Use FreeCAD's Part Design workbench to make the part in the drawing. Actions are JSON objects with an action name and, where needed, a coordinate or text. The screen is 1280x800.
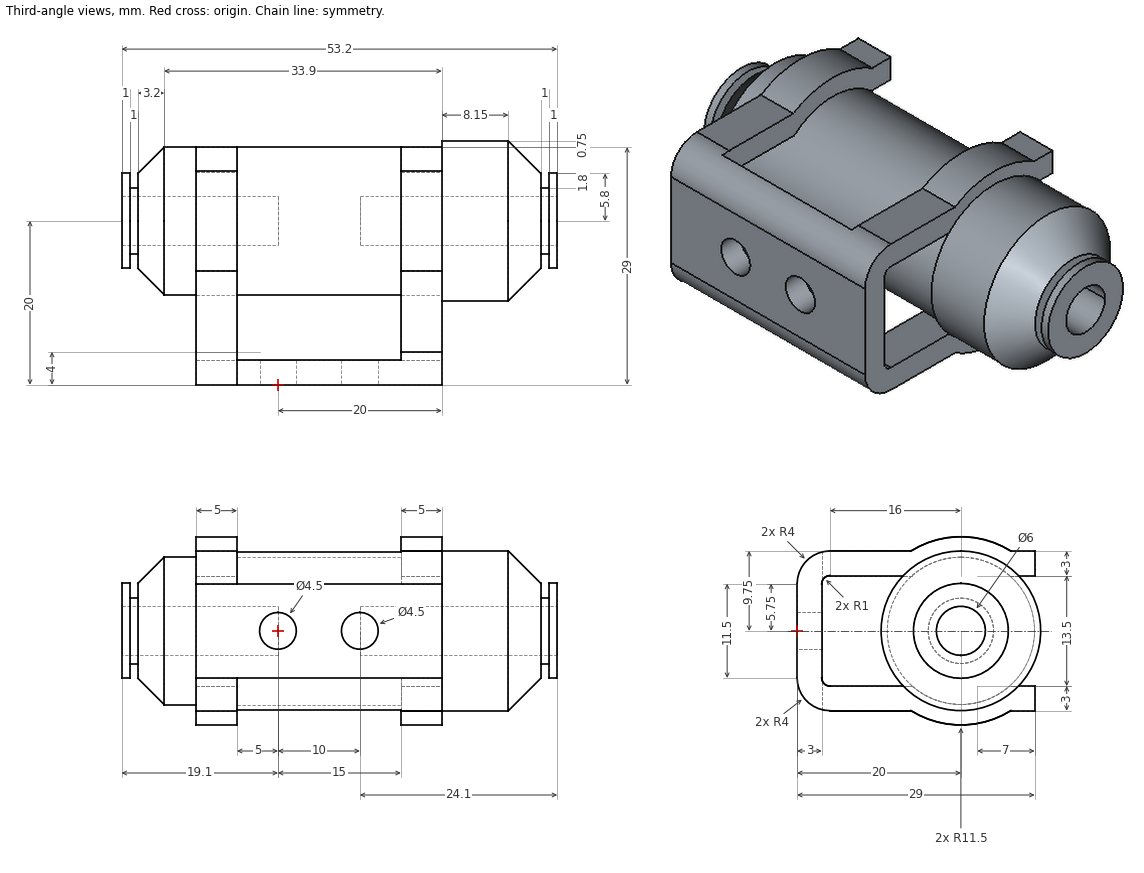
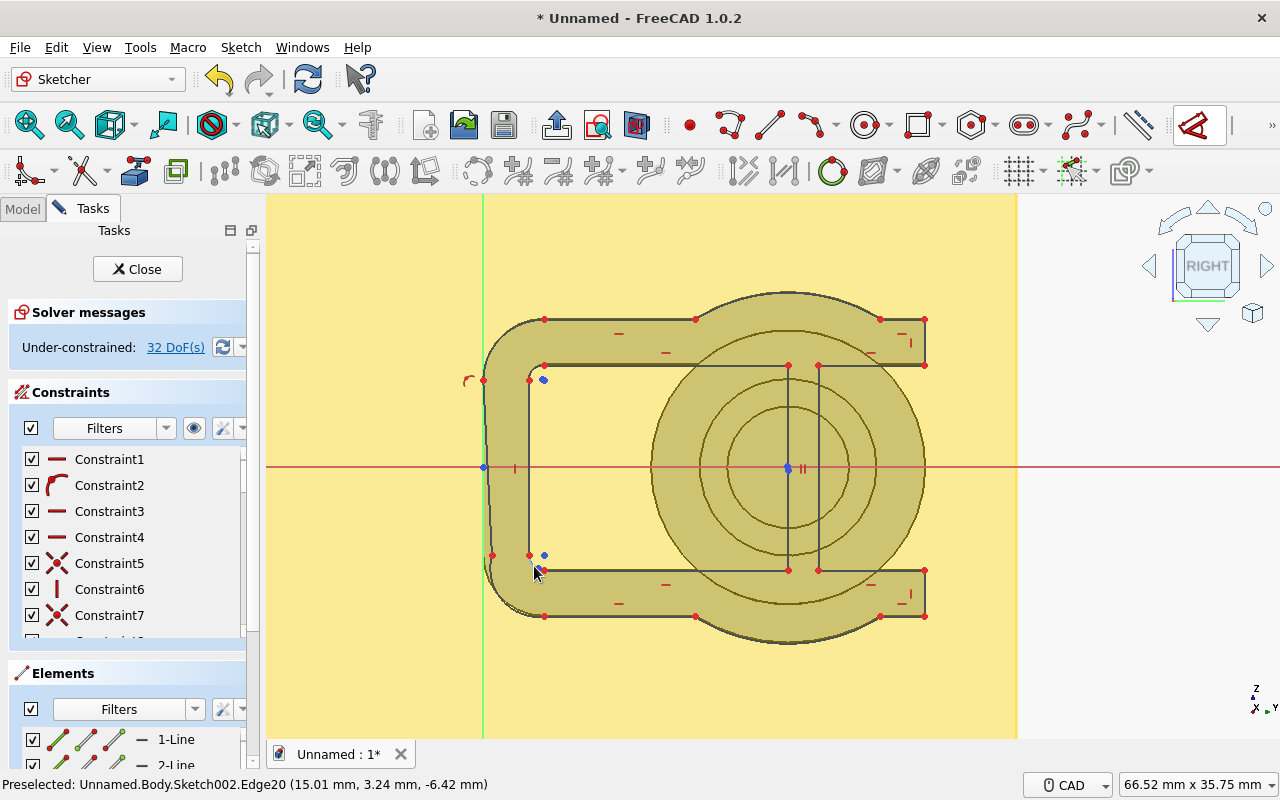
{"action": "left_click", "coordinate": [650, 320]}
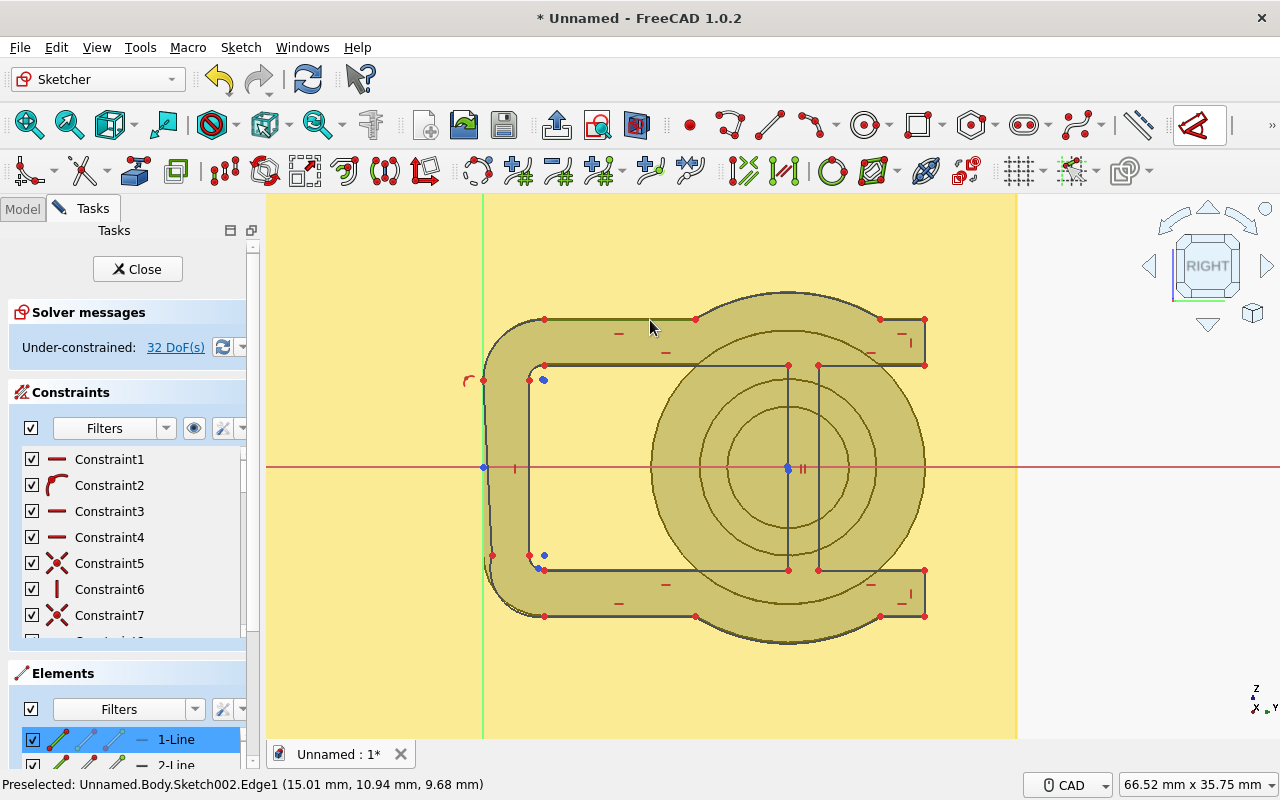
{"action": "left_click", "coordinate": [516, 326]}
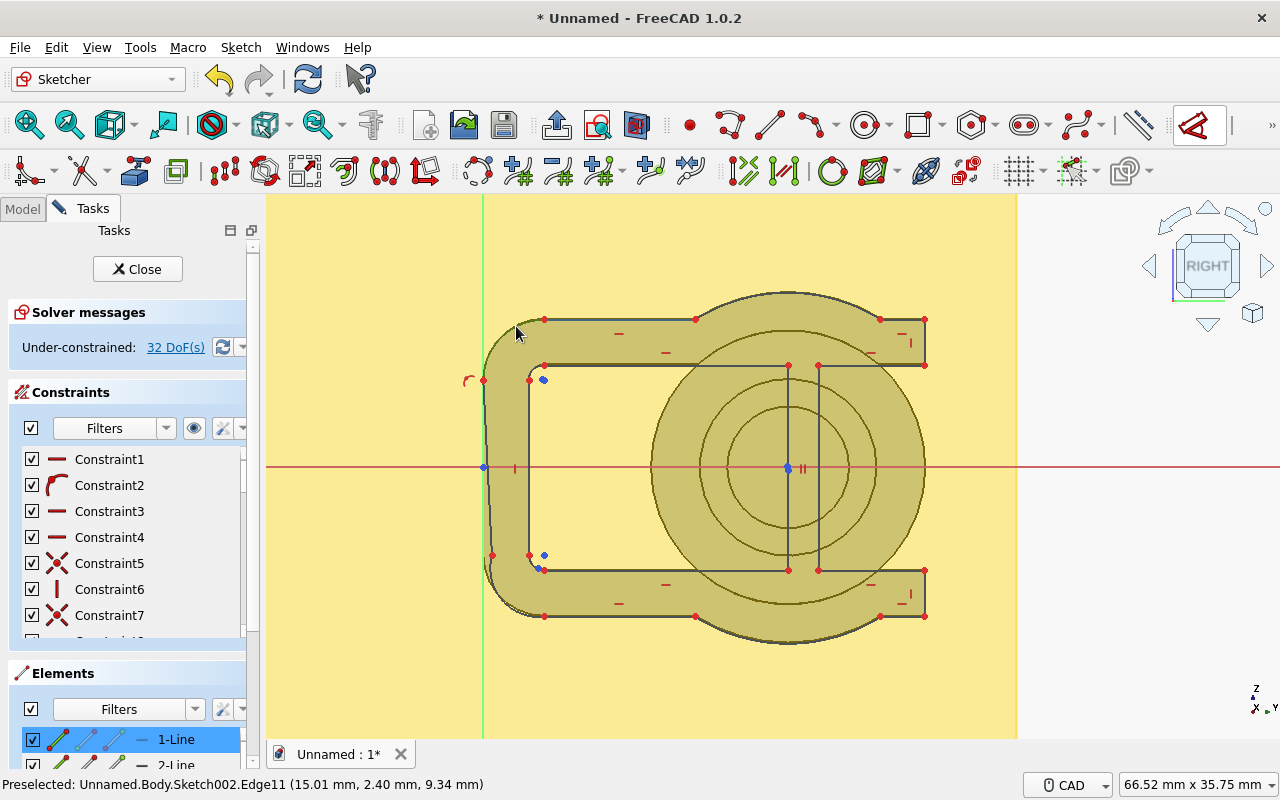
{"action": "key", "text": "t"}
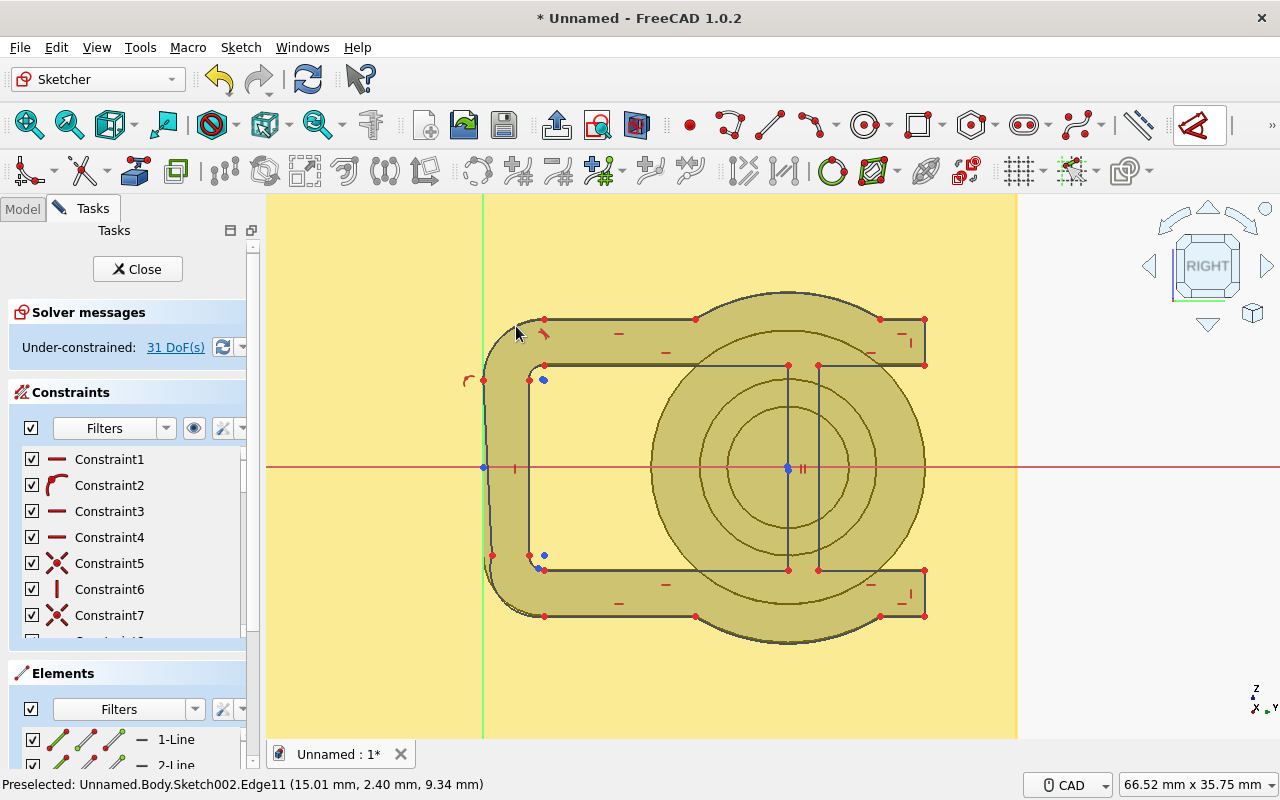
{"action": "left_click", "coordinate": [486, 433]}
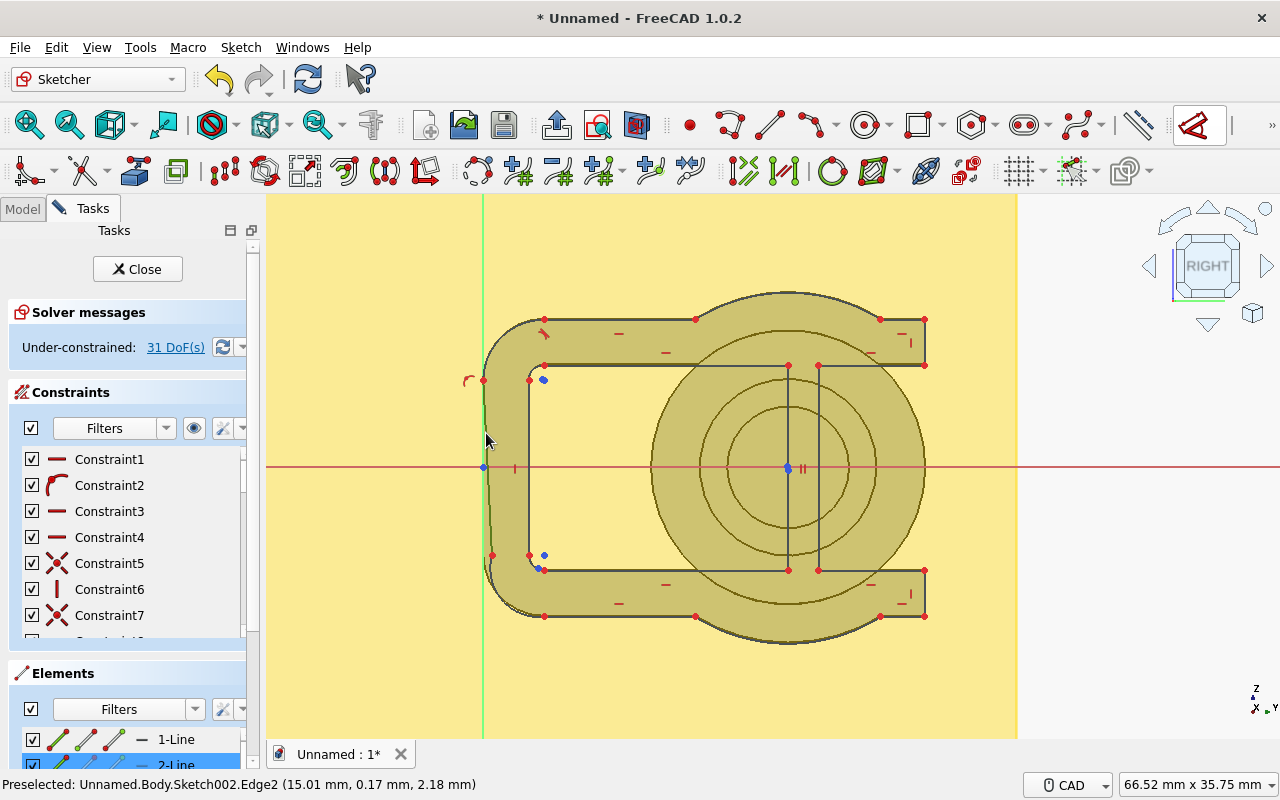
{"action": "left_click", "coordinate": [517, 326]}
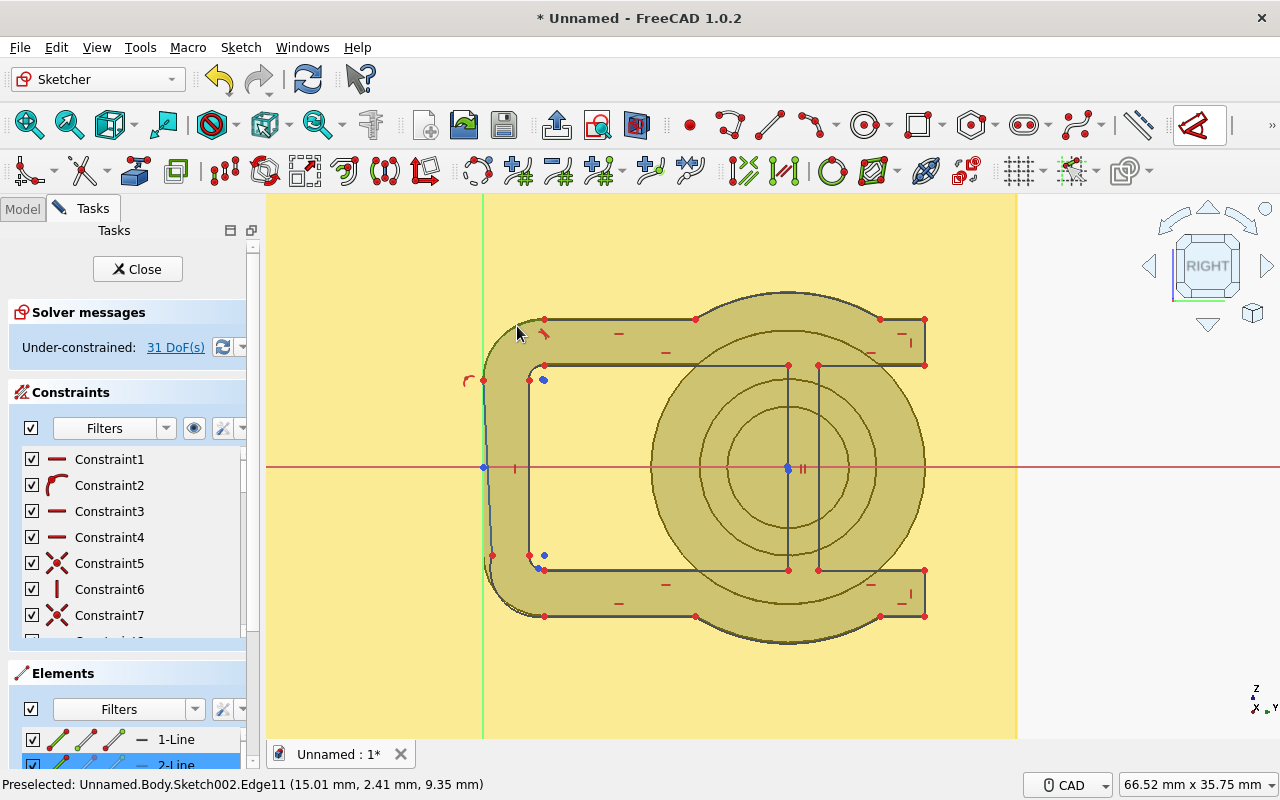
{"action": "key", "text": "t"}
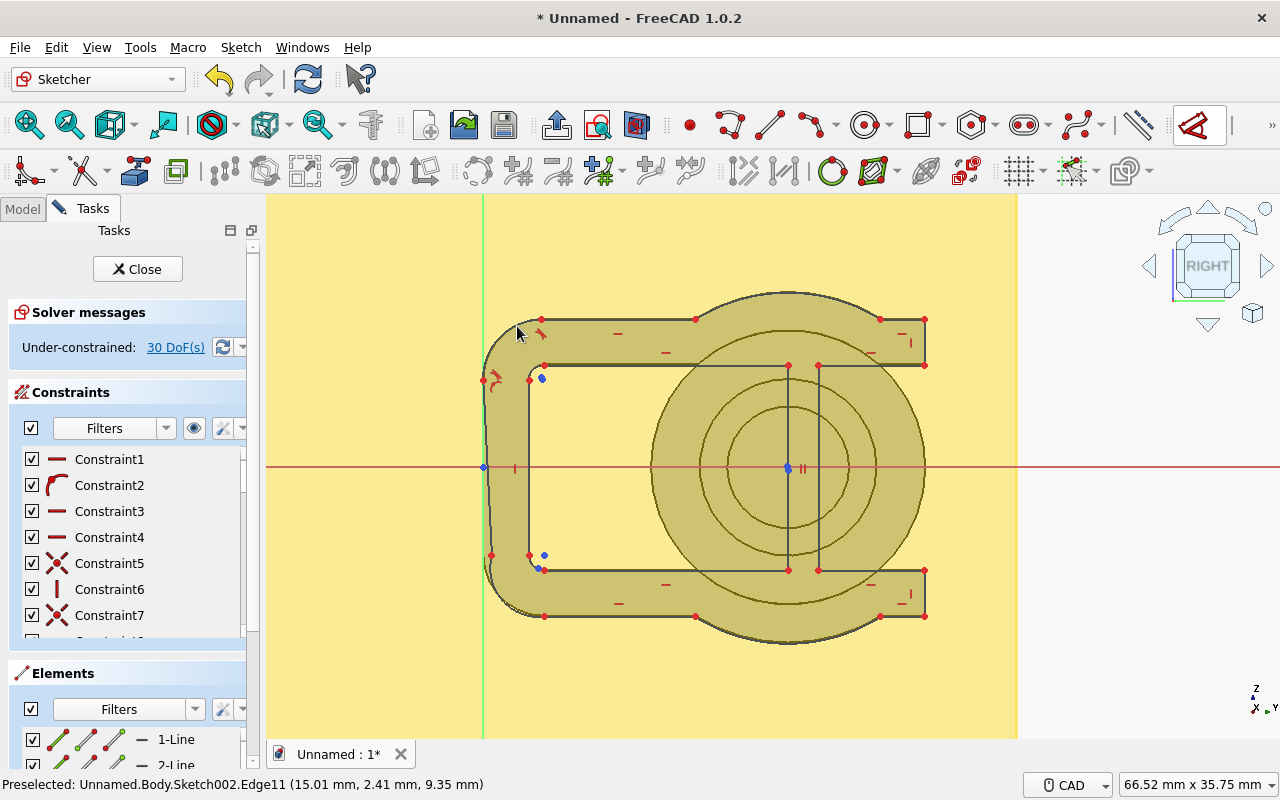
{"action": "left_click", "coordinate": [486, 433]}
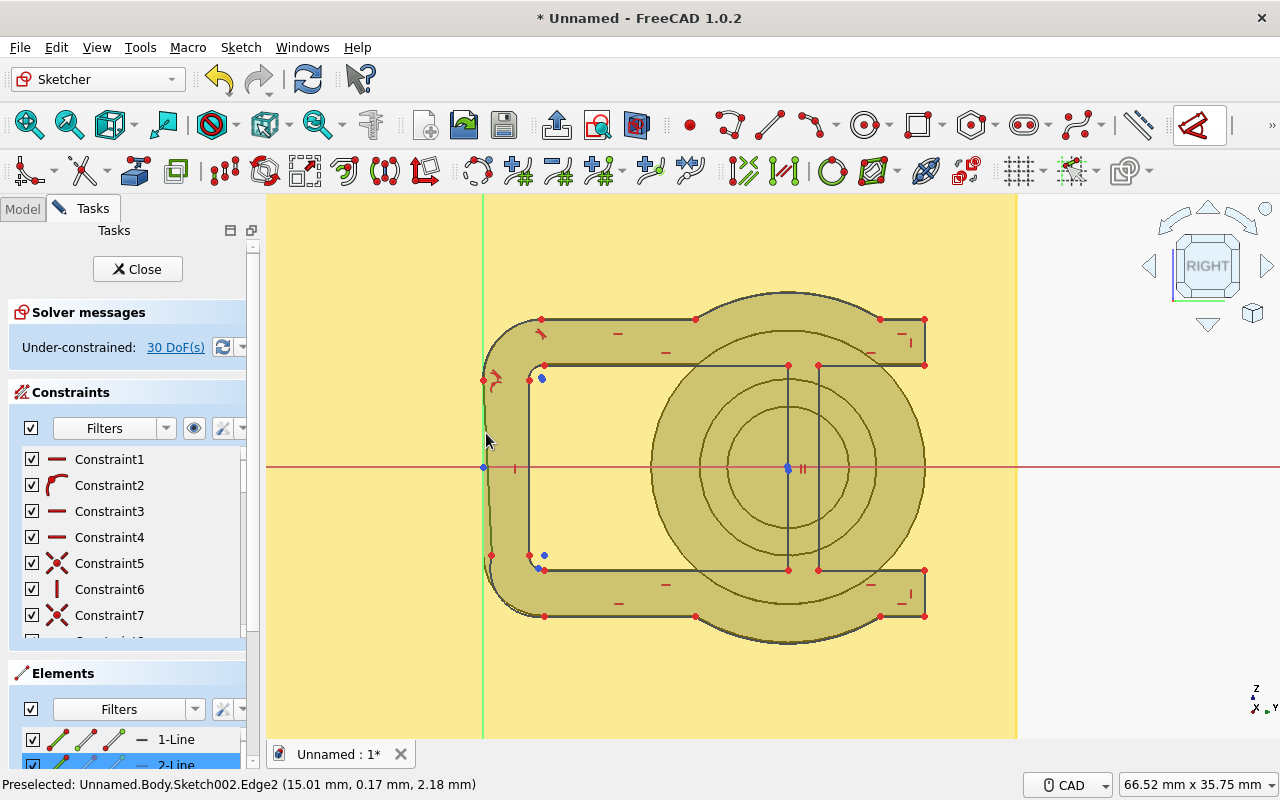
{"action": "scroll", "coordinate": [493, 584], "scroll_direction": "up", "scroll_amount": 2}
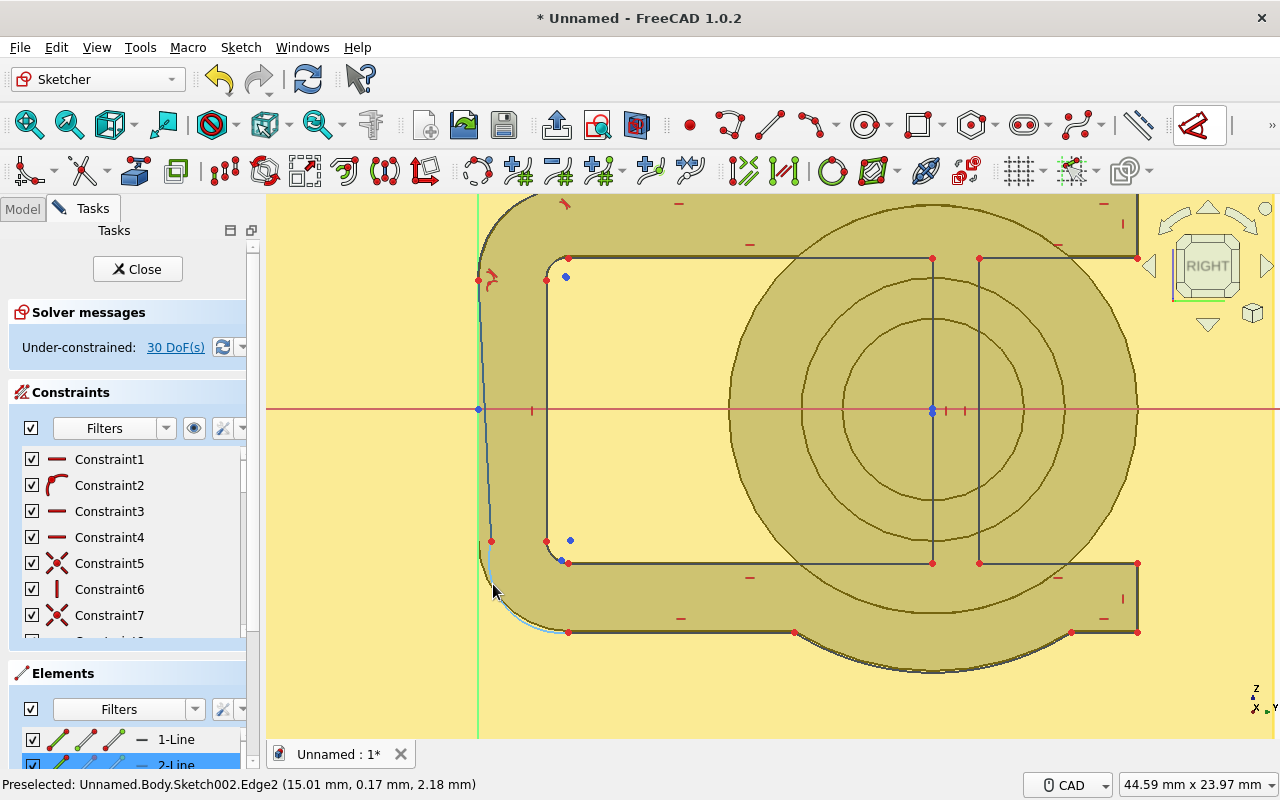
{"action": "left_click", "coordinate": [493, 583]}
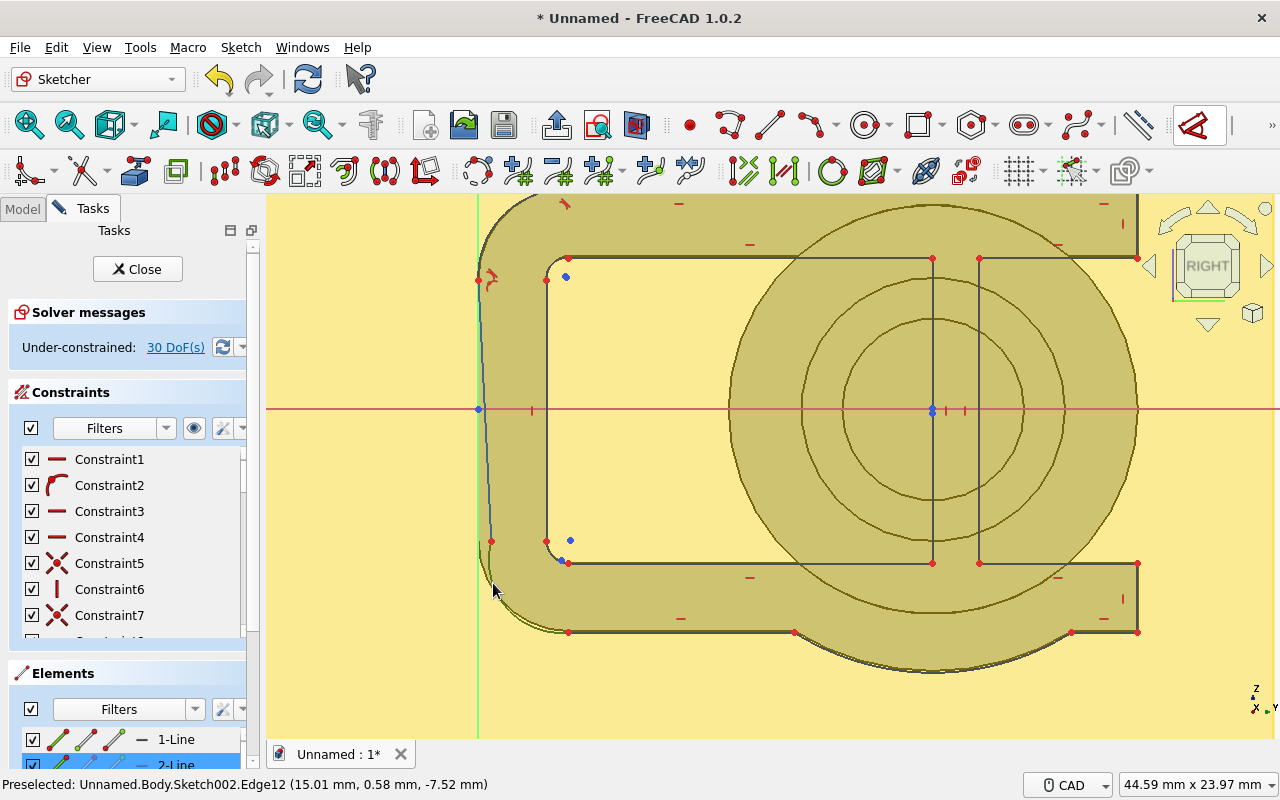
{"action": "key", "text": "t"}